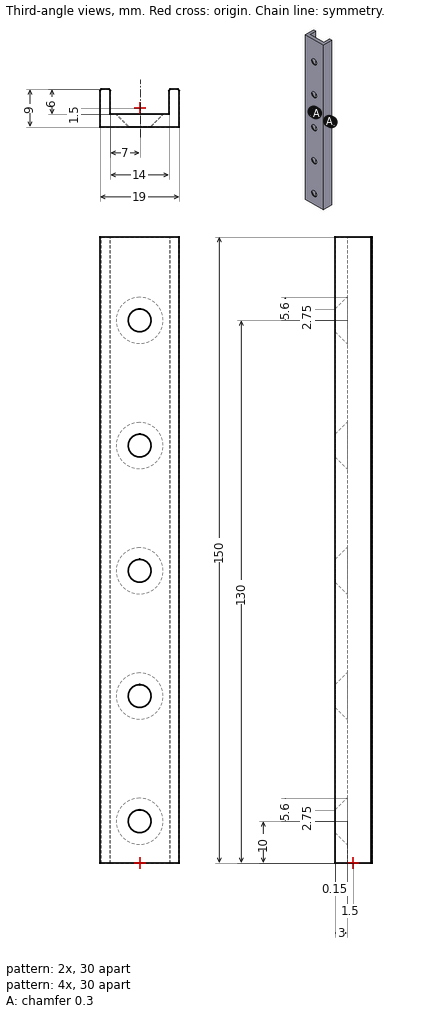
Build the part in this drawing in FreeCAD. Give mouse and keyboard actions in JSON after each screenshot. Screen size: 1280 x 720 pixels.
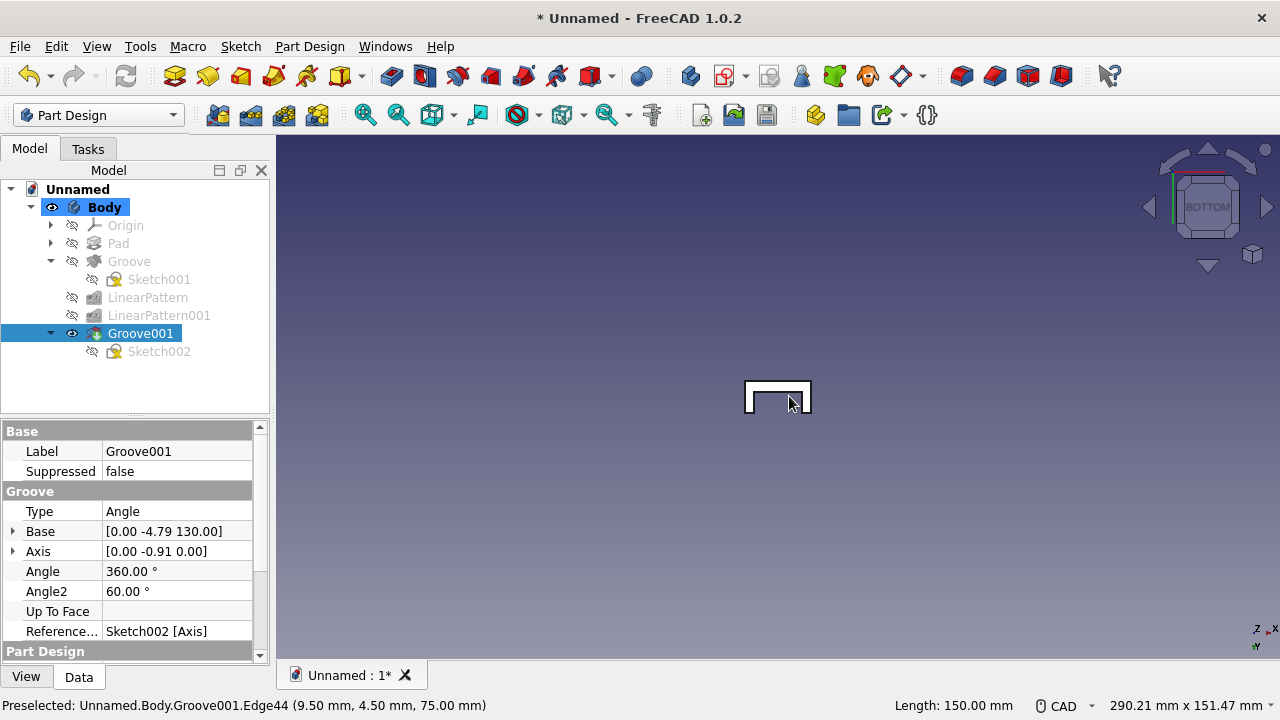
{"action": "left_click", "coordinate": [366, 116]}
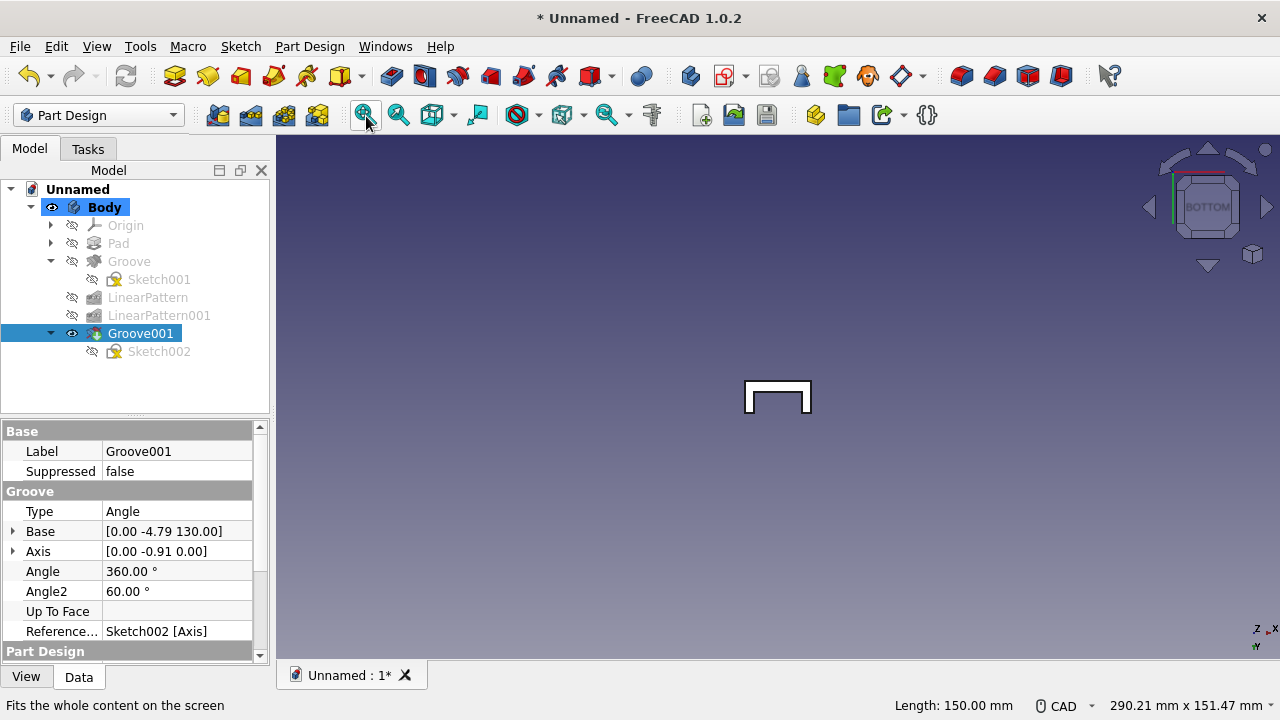
{"action": "key", "text": "4"}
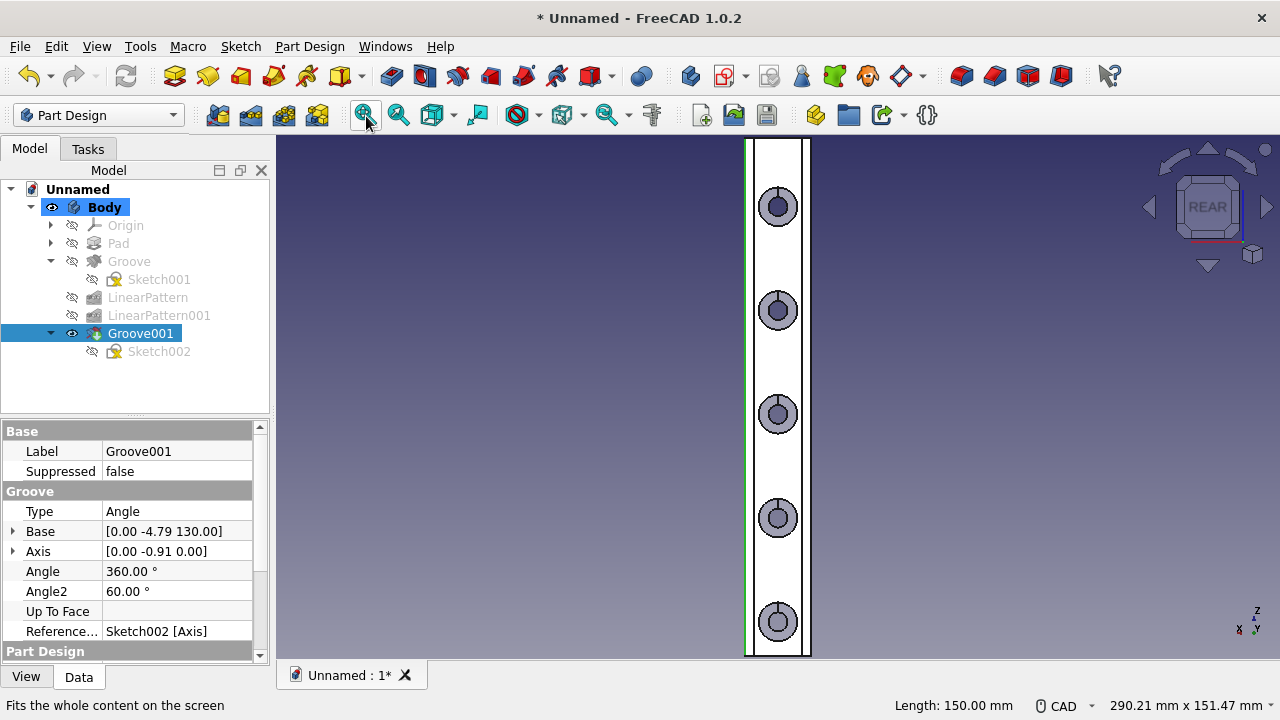
{"action": "left_click", "coordinate": [811, 396], "text": "ctrl"}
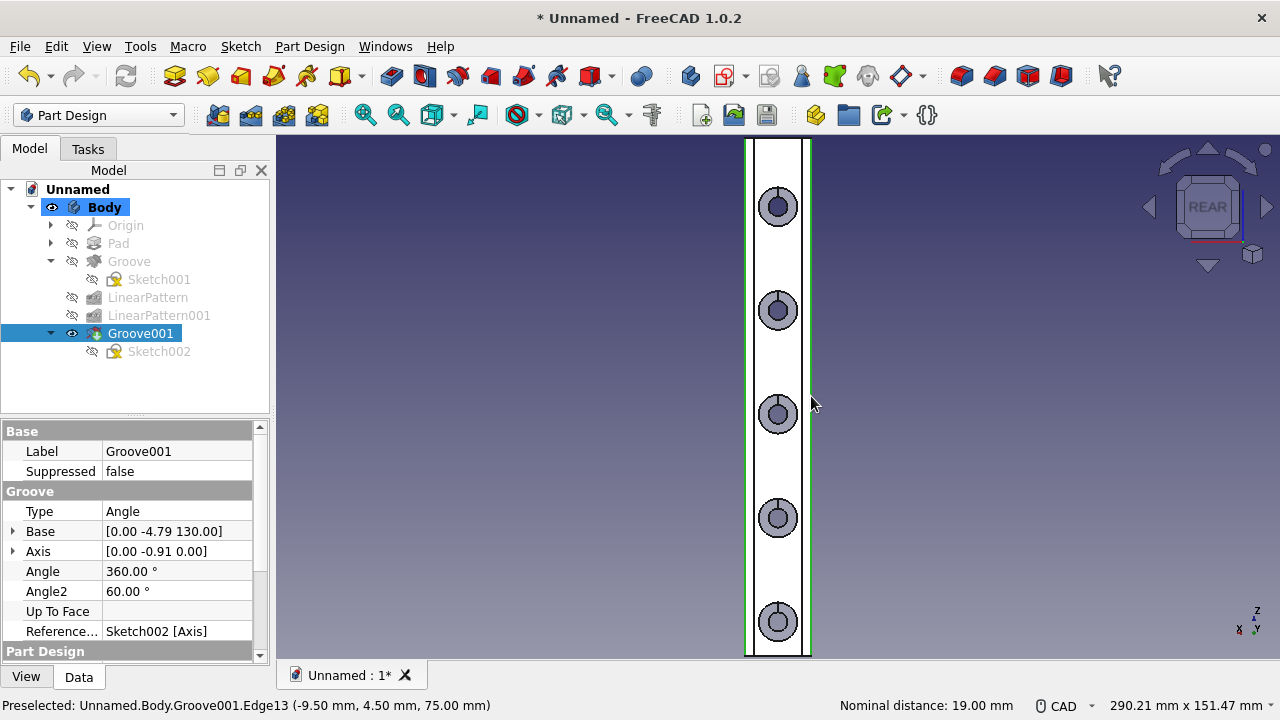
{"action": "left_click", "coordinate": [802, 396], "text": "ctrl"}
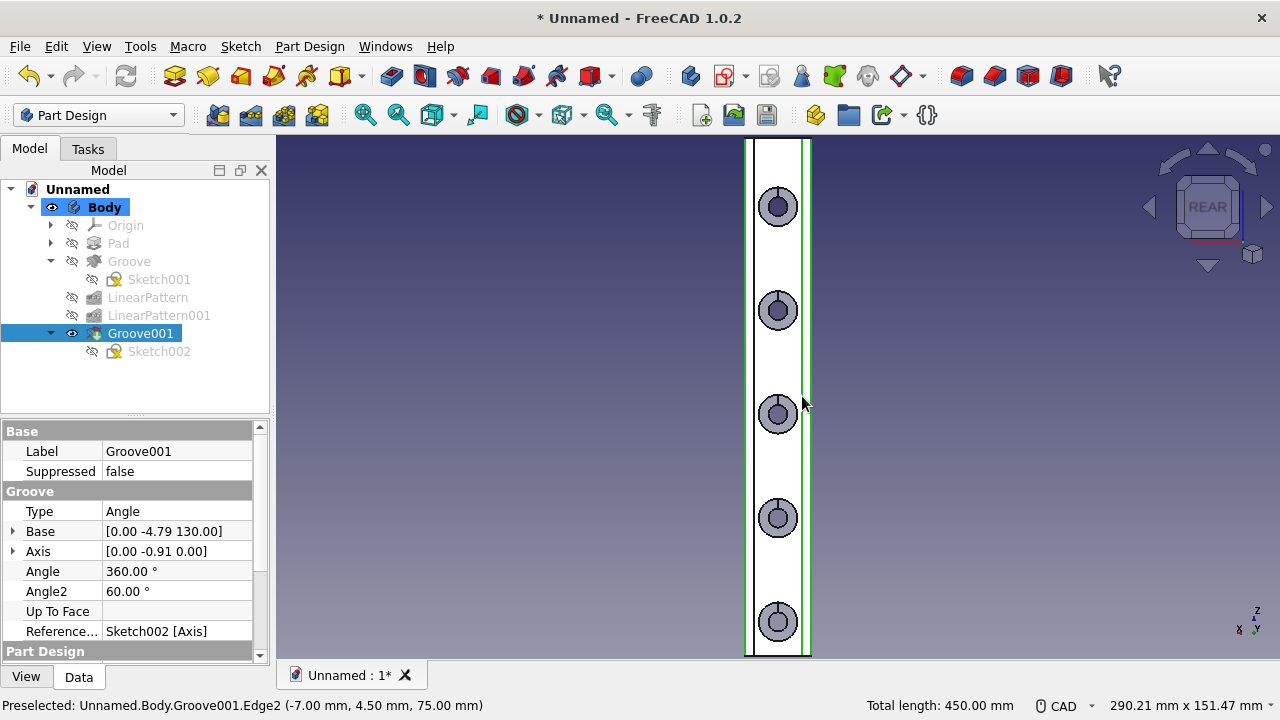
{"action": "left_click", "coordinate": [754, 396], "text": "ctrl"}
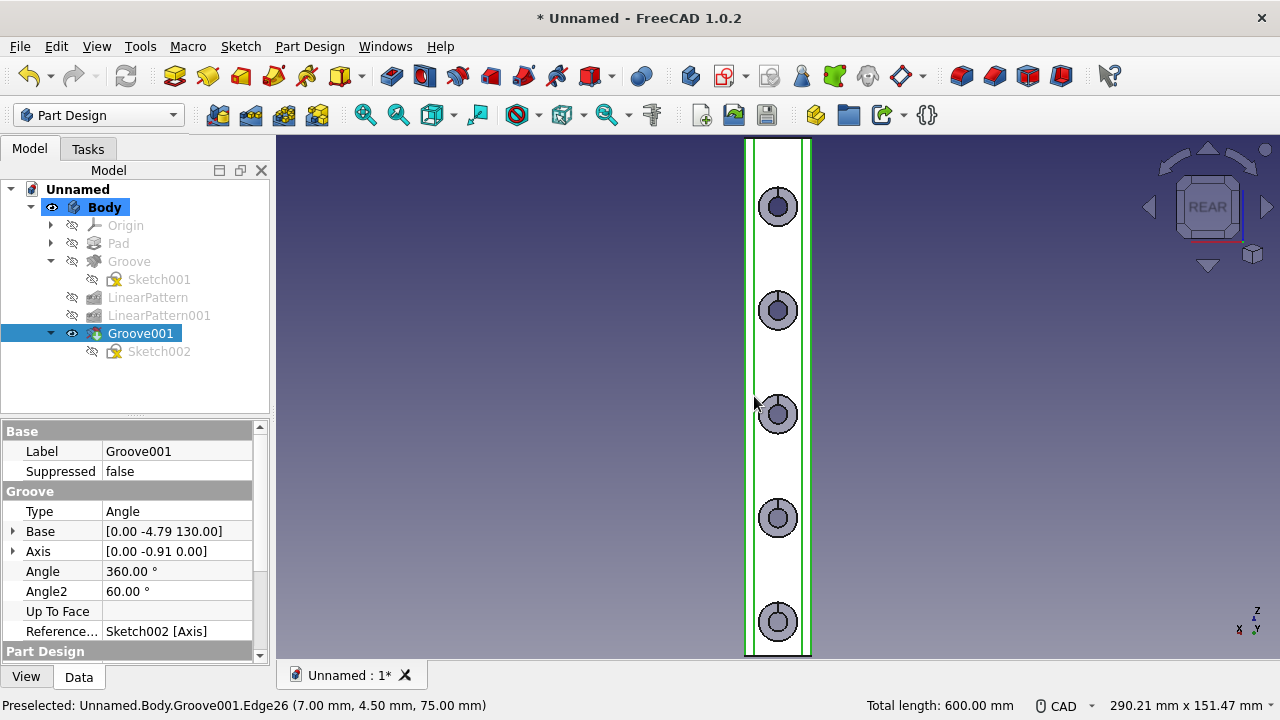
{"action": "left_click", "coordinate": [995, 76]}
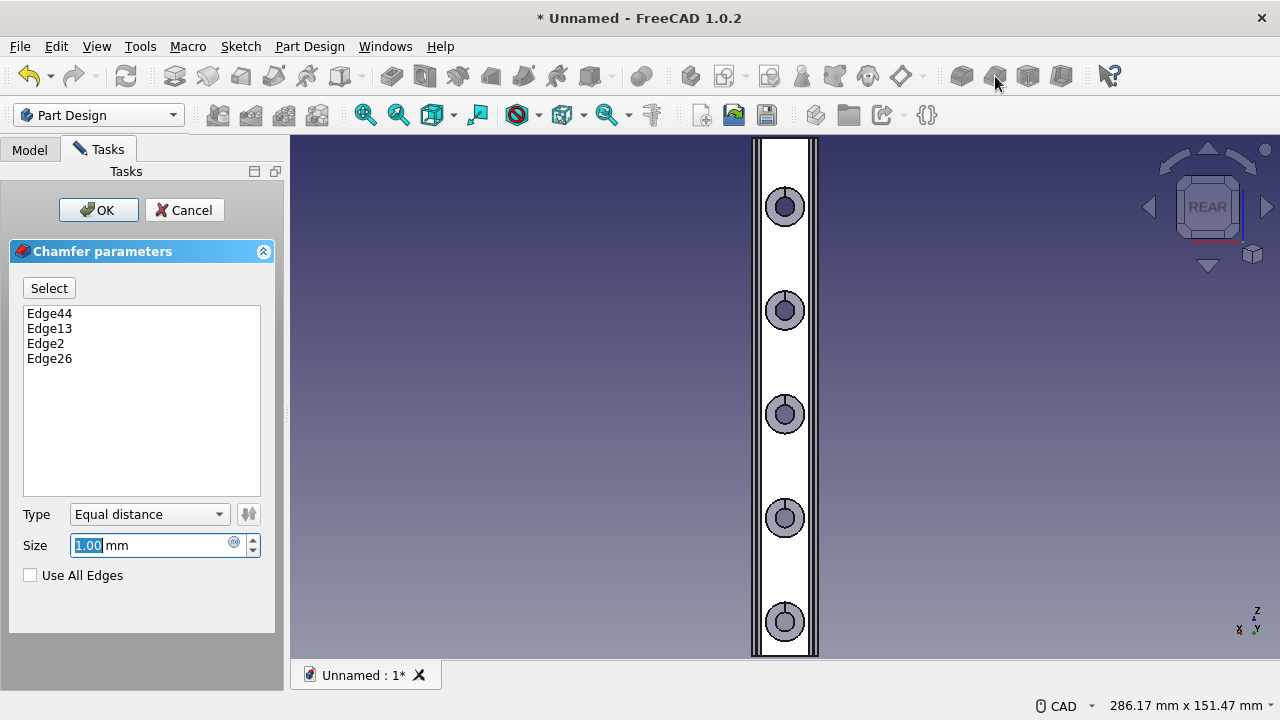
{"action": "type", "text": "0.3"}
{"action": "key", "text": "Tab"}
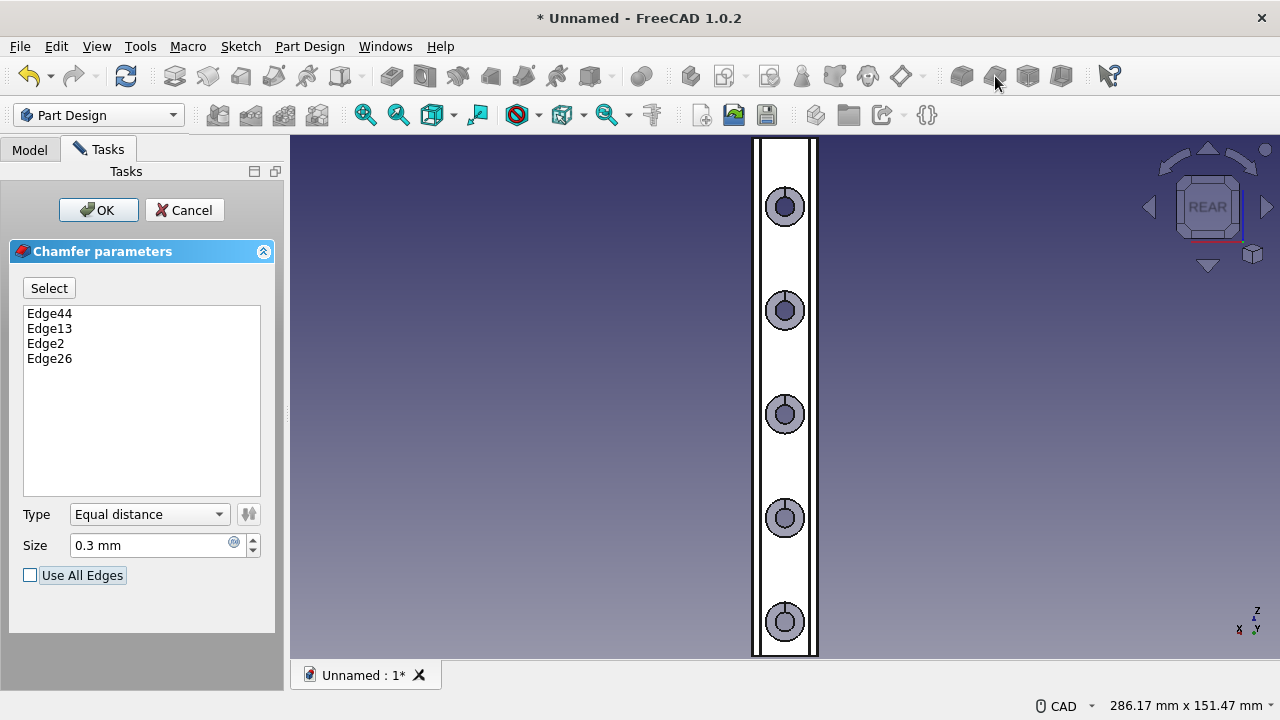
{"action": "left_click", "coordinate": [99, 210]}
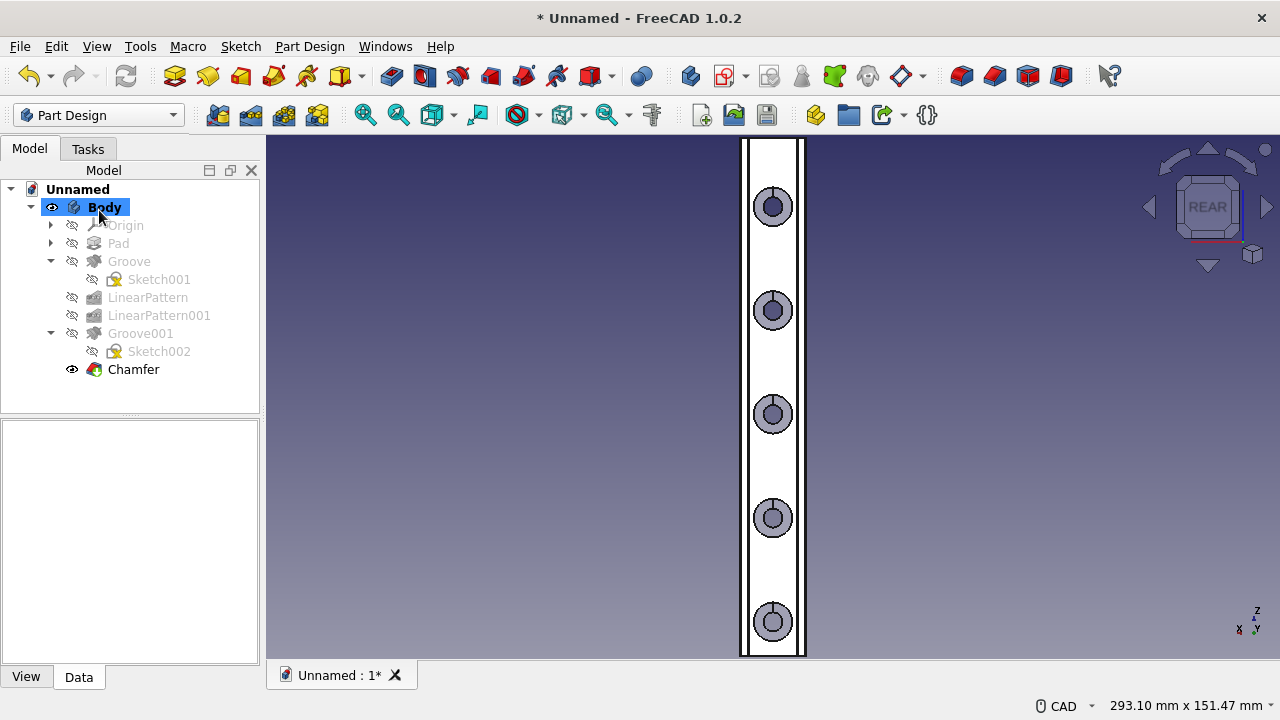
{"action": "key", "text": "0"}